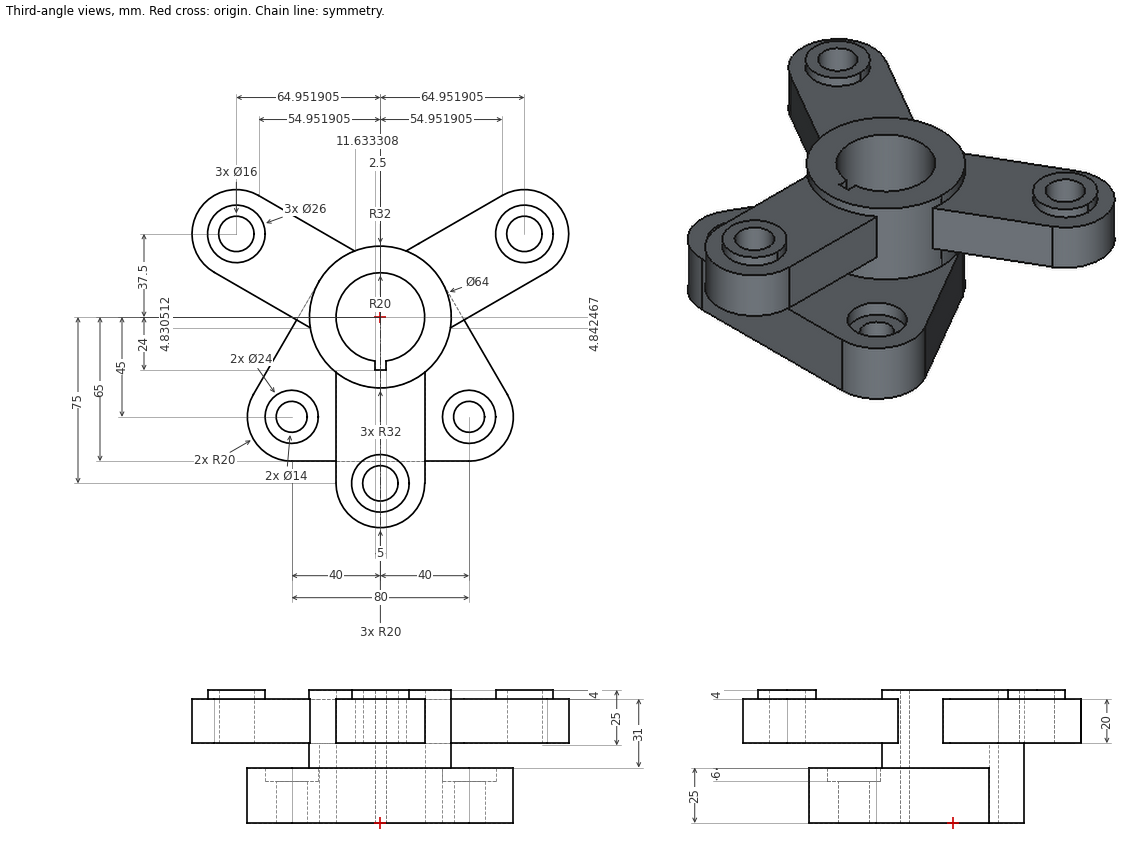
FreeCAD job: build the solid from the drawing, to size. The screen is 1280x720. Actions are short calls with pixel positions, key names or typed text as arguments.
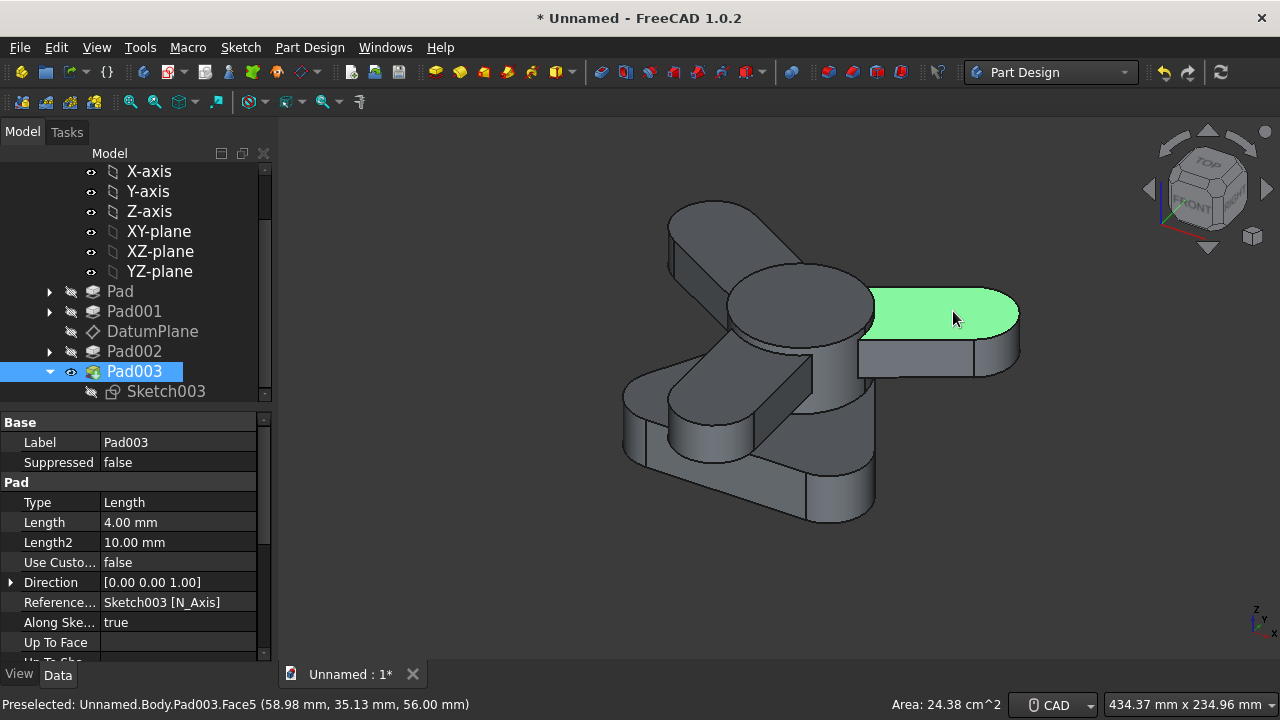
click(168, 72)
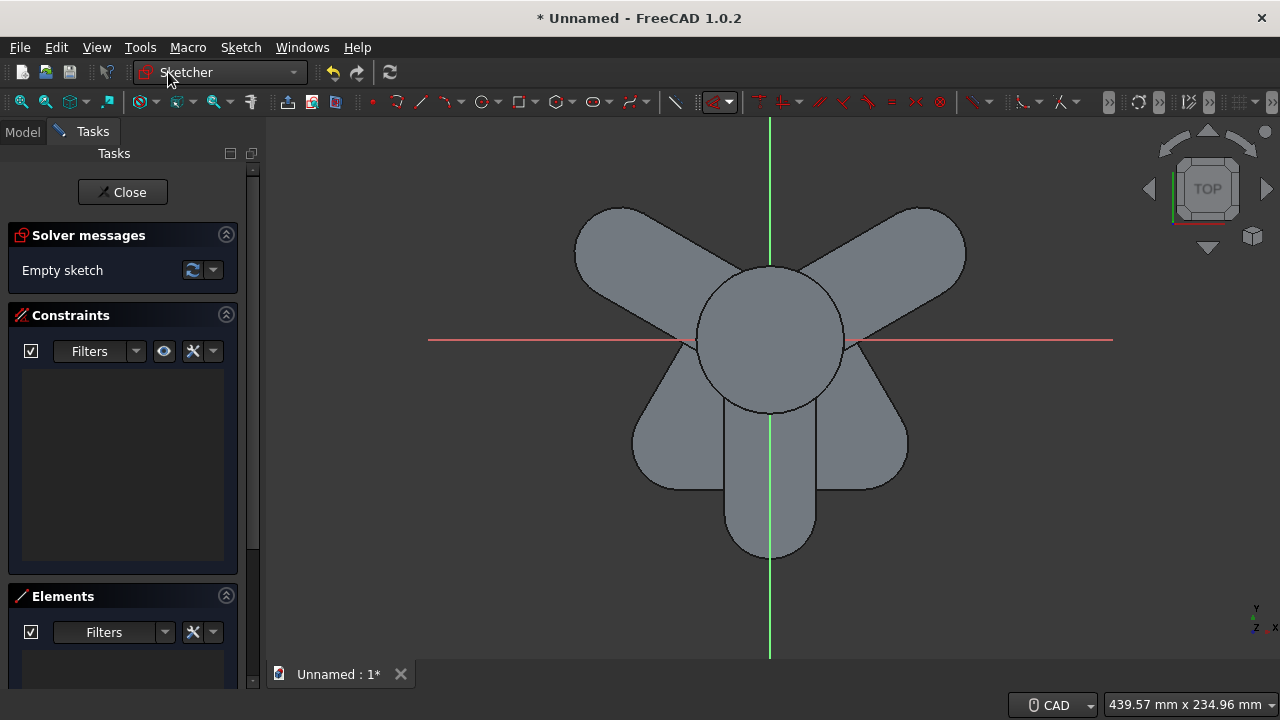
key(g)
key(c)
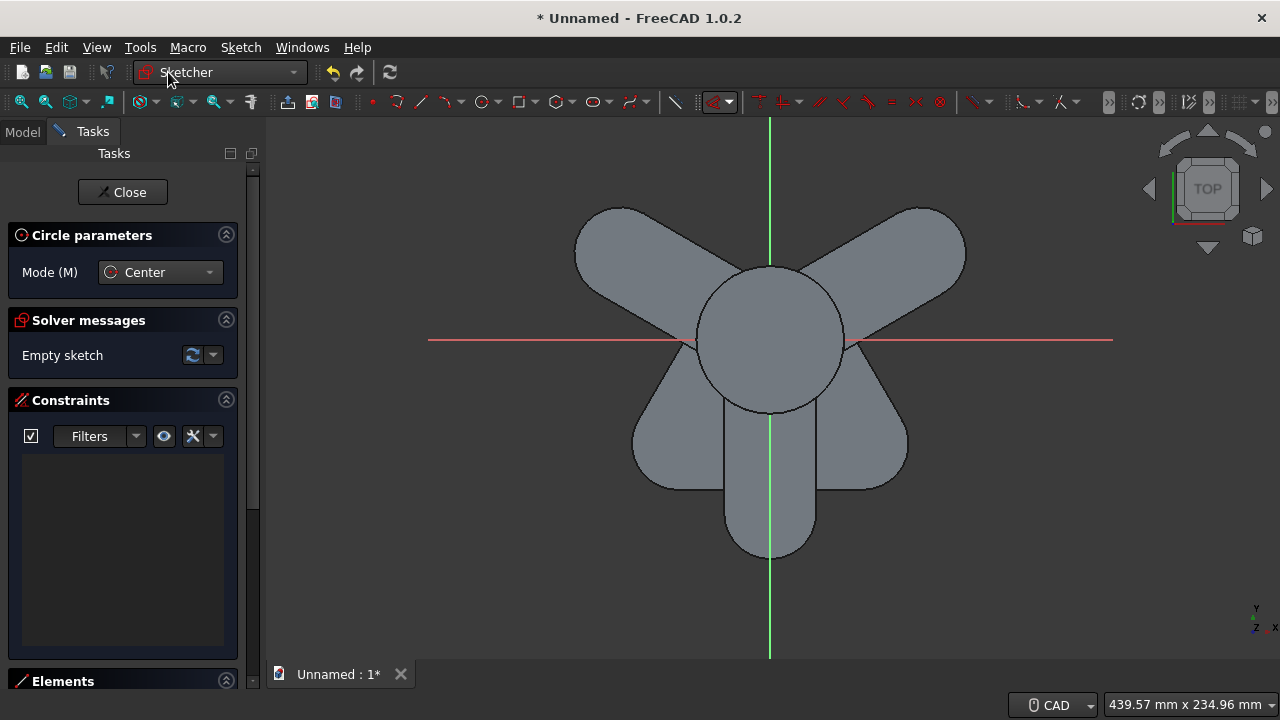
click(620, 253)
click(642, 232)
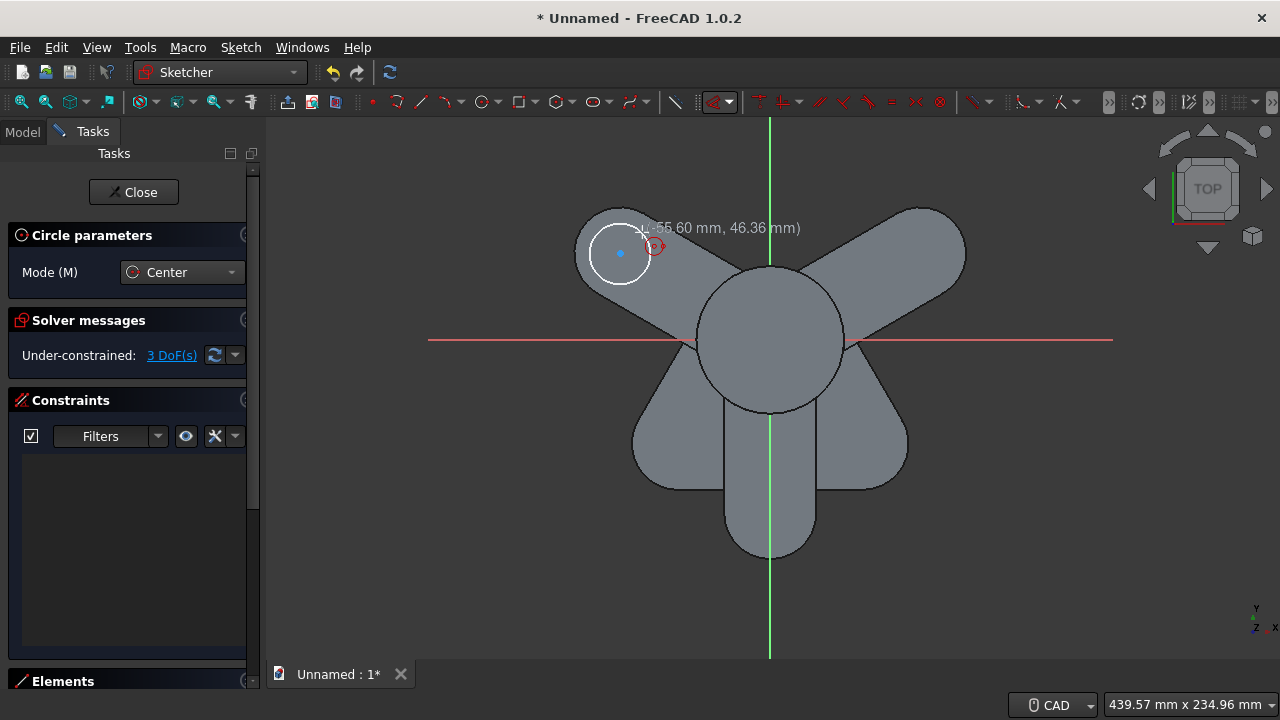
click(920, 253)
click(941, 232)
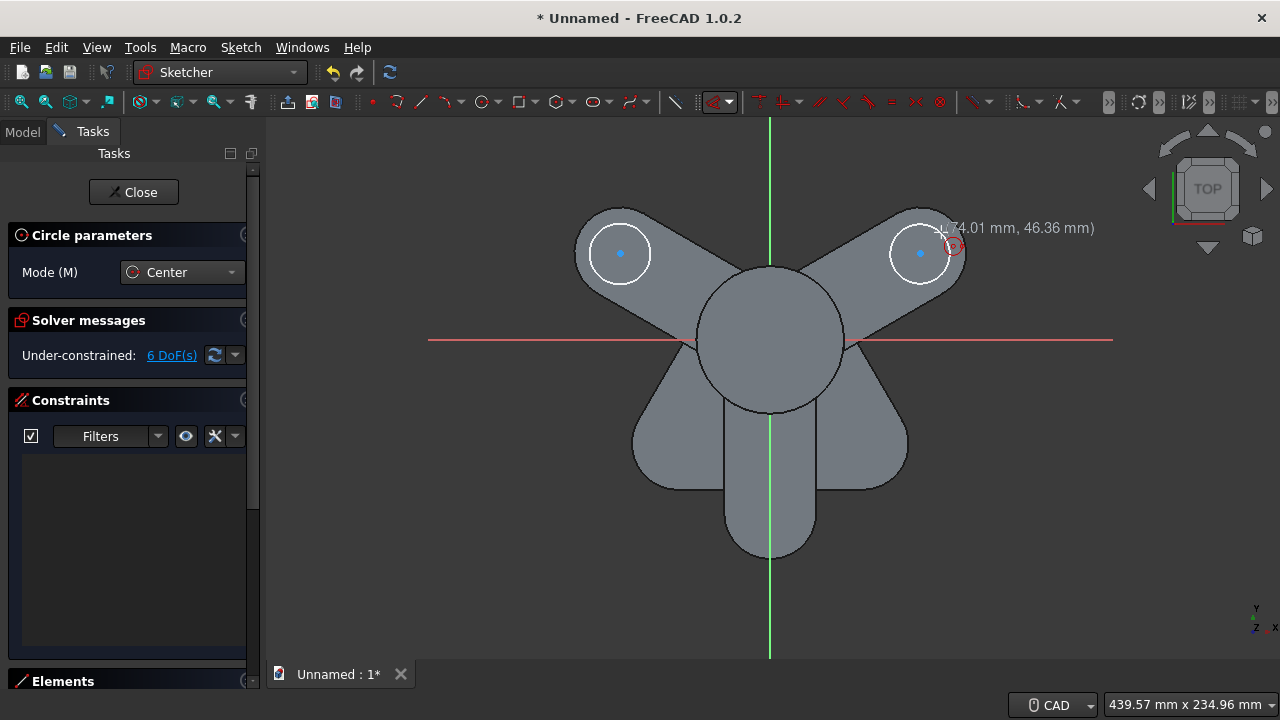
click(770, 513)
click(791, 492)
key(Escape)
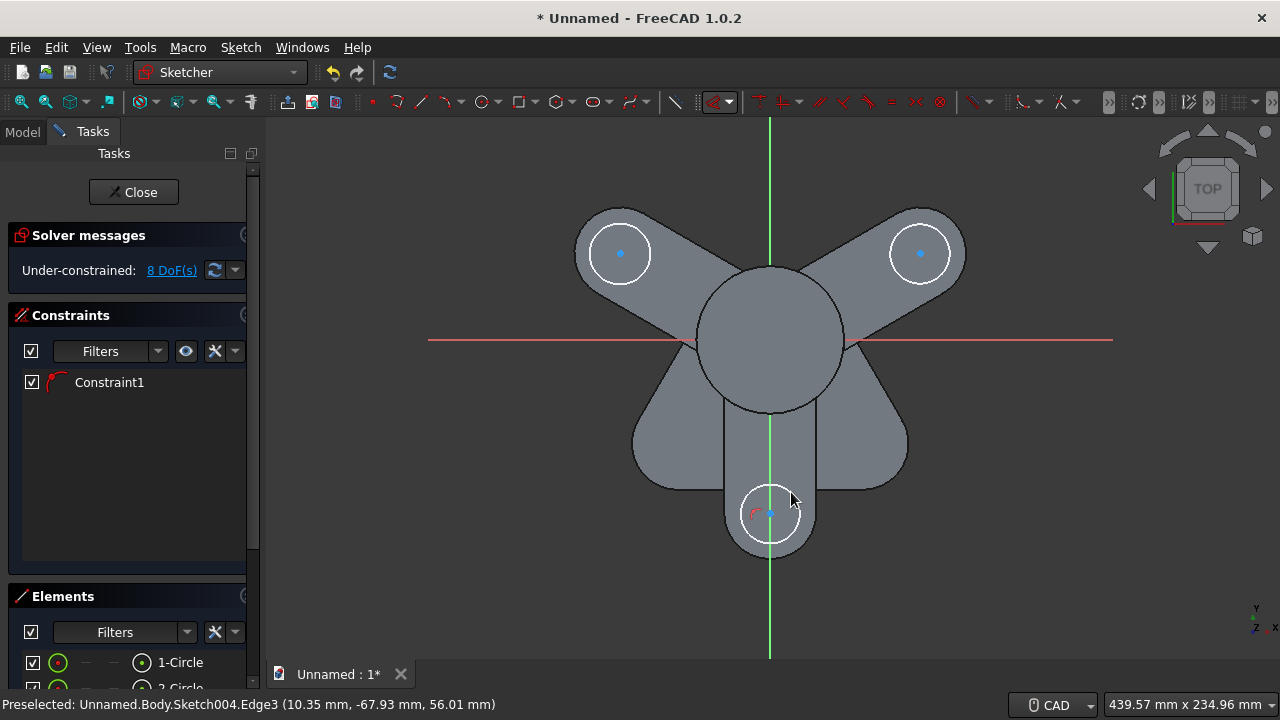
click(641, 232)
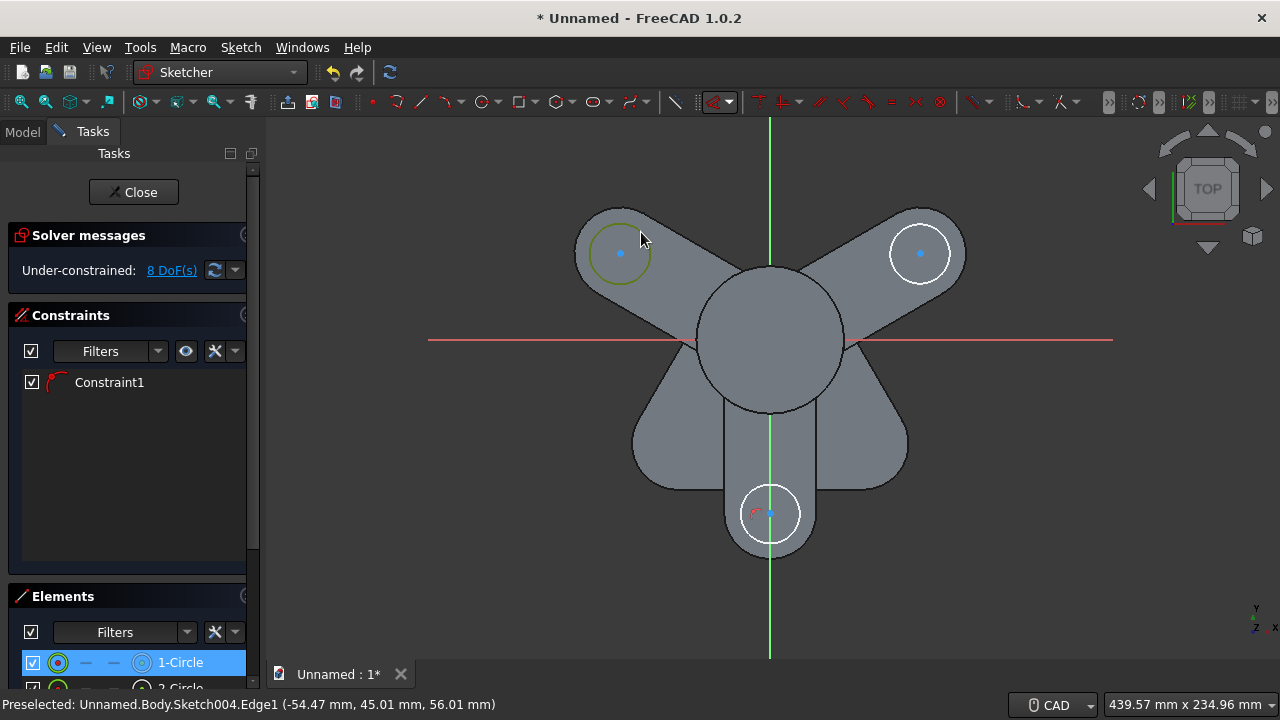
click(941, 233)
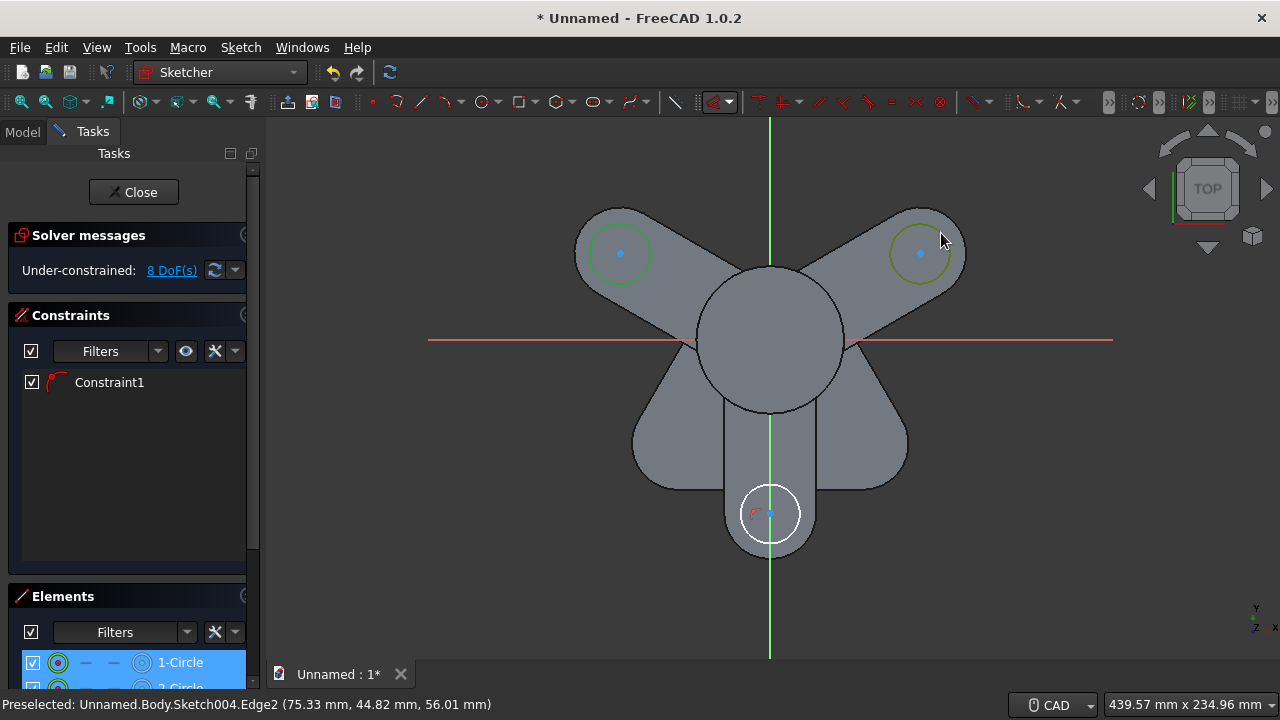
click(791, 493)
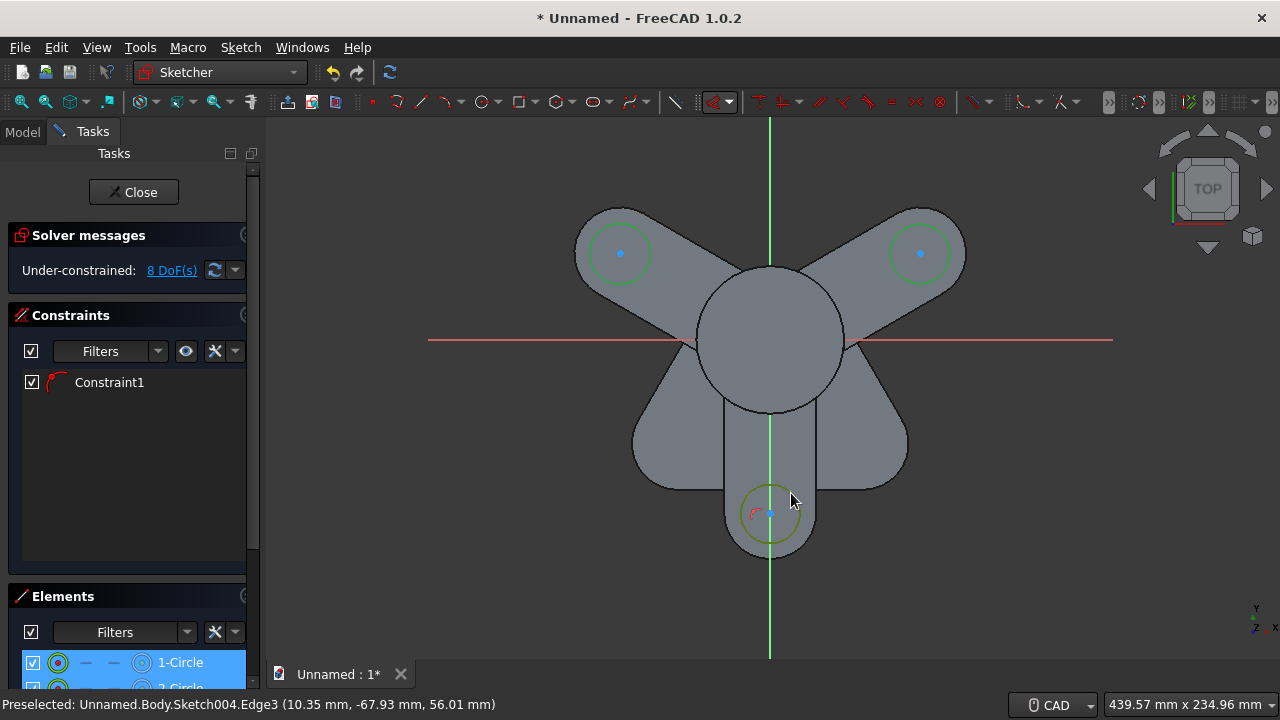
key(e)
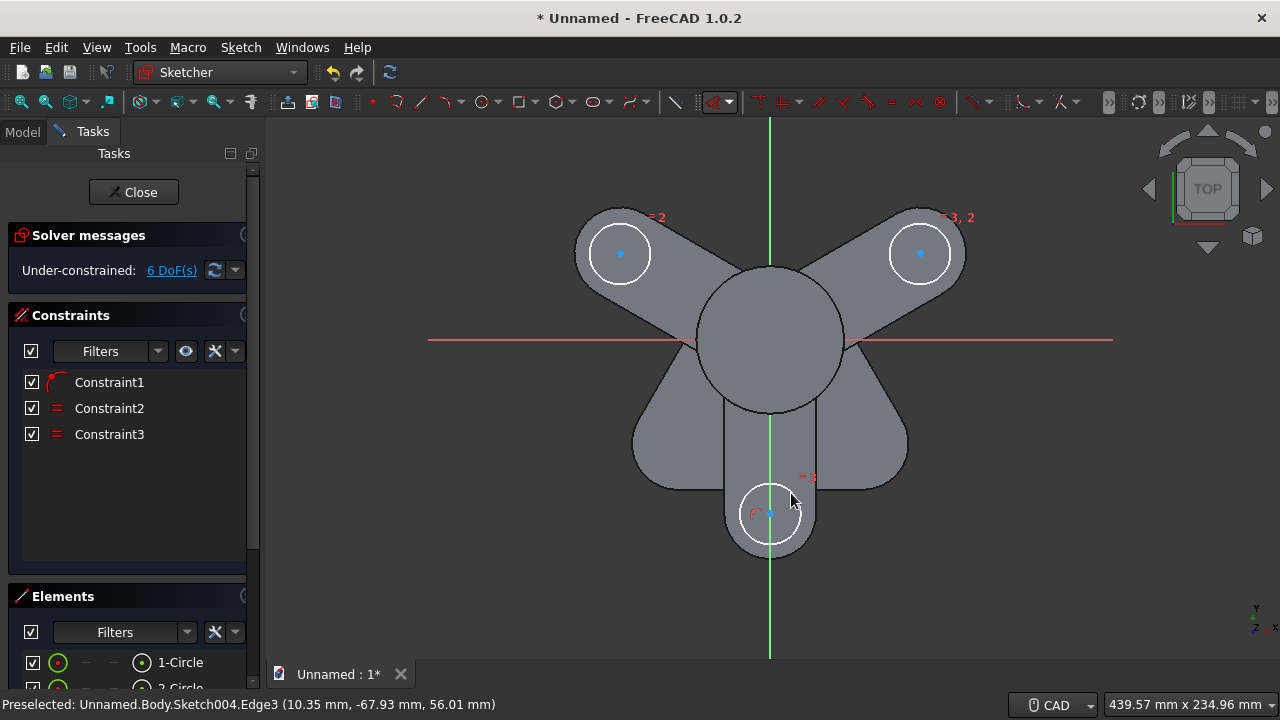
click(620, 254)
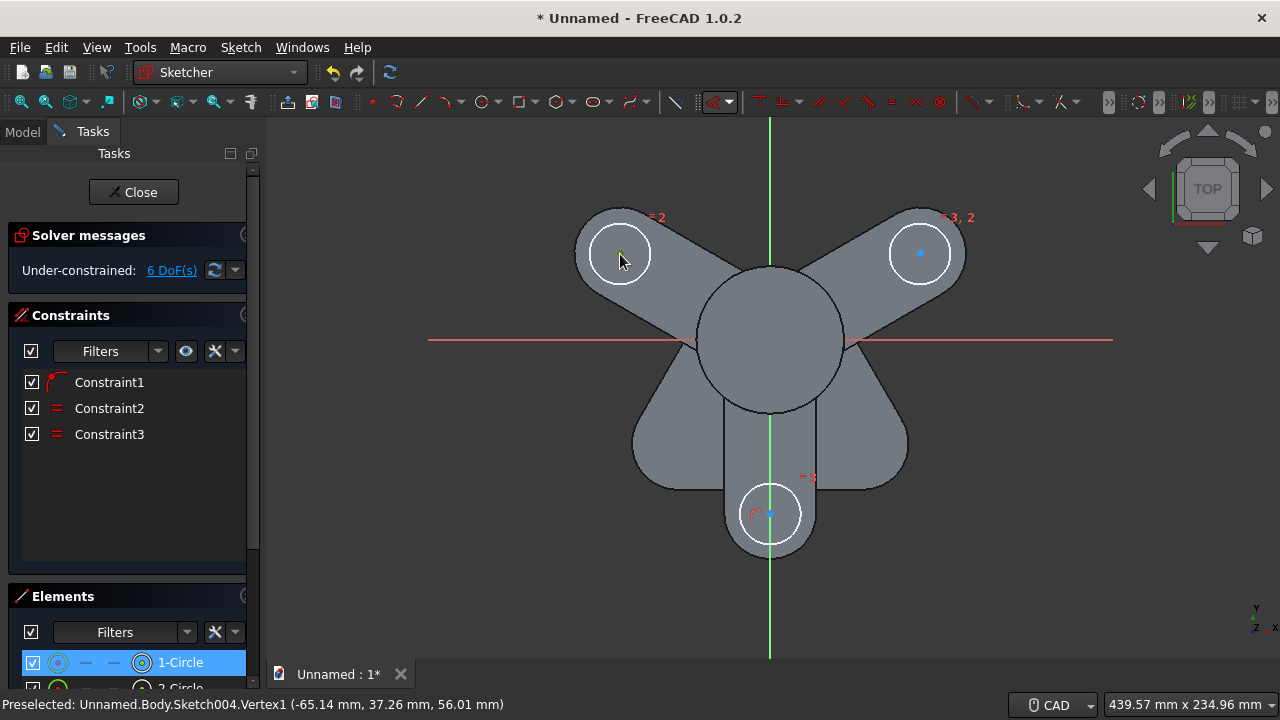
click(920, 254)